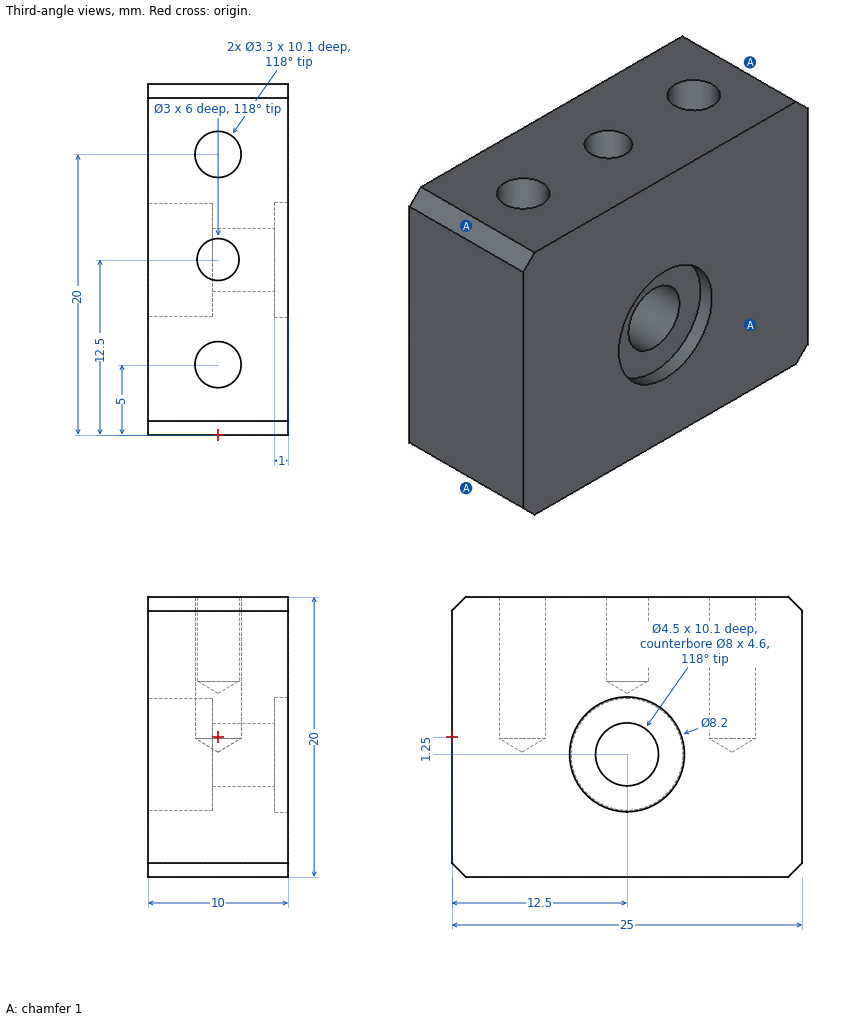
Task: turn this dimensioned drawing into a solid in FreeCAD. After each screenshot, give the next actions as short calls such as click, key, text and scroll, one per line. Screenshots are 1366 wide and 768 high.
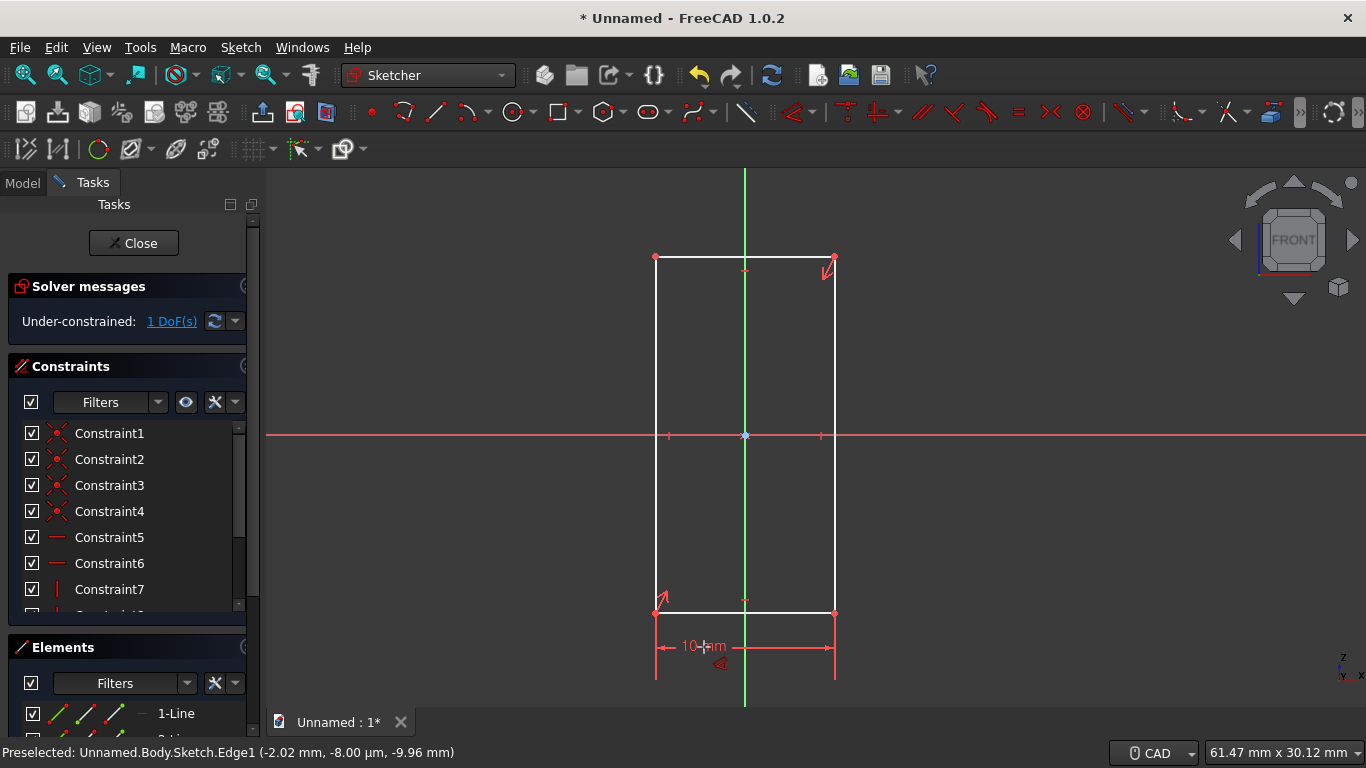
click(835, 506)
click(869, 353)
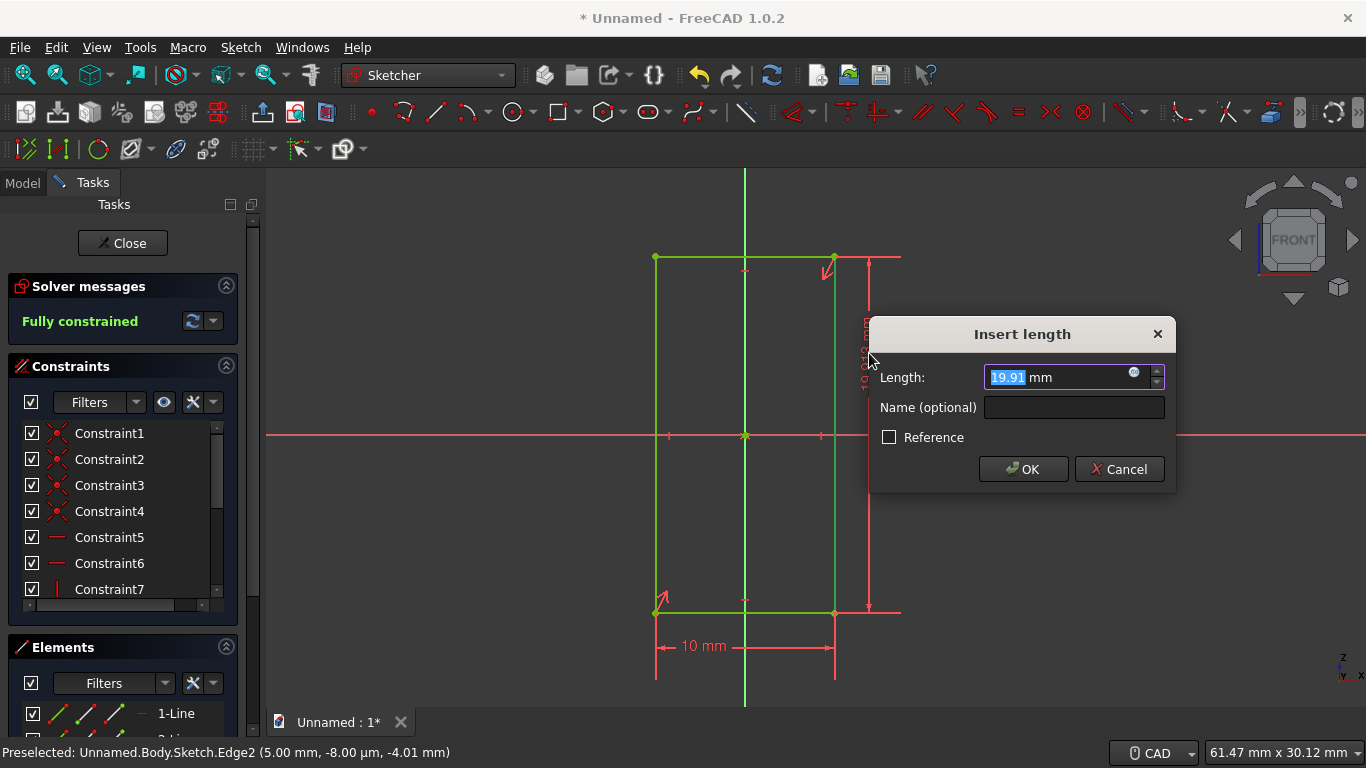
text(20)
key(Return)
key(Escape)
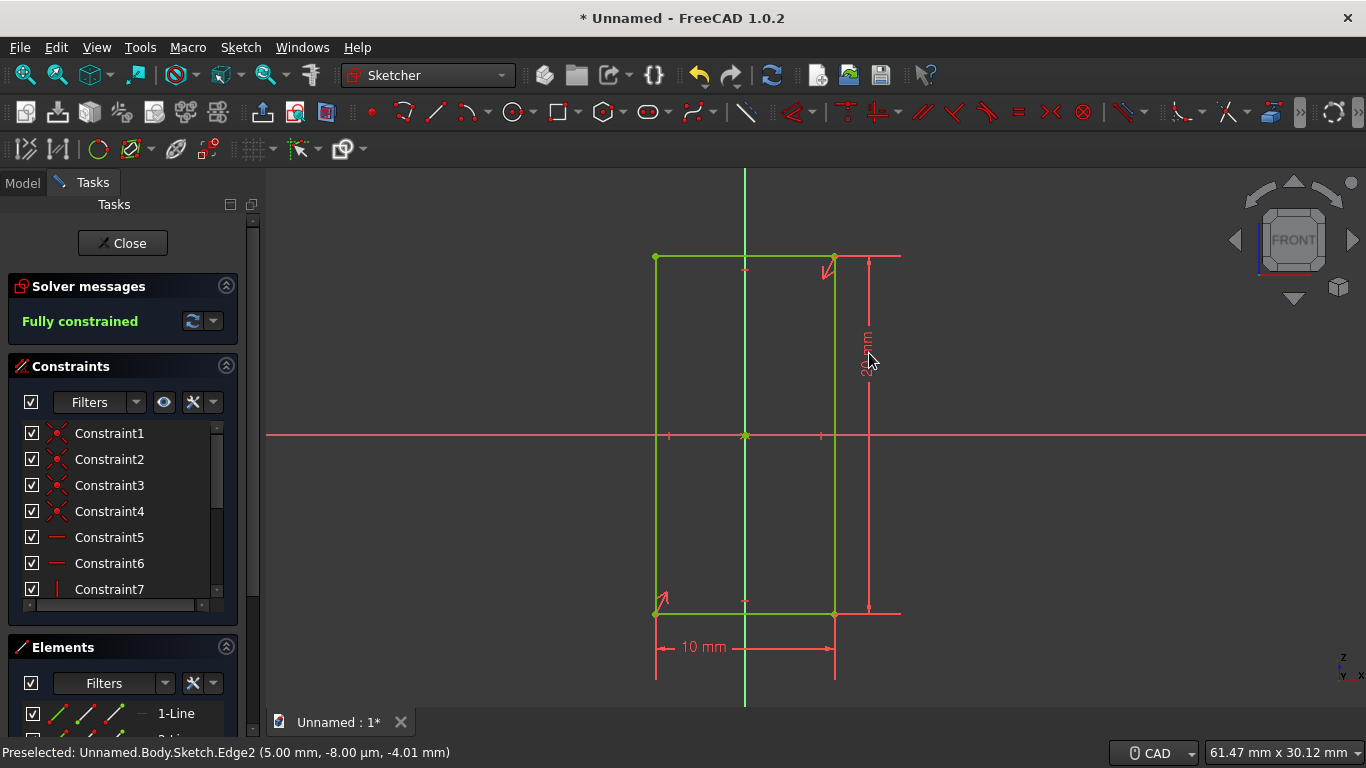
click(123, 243)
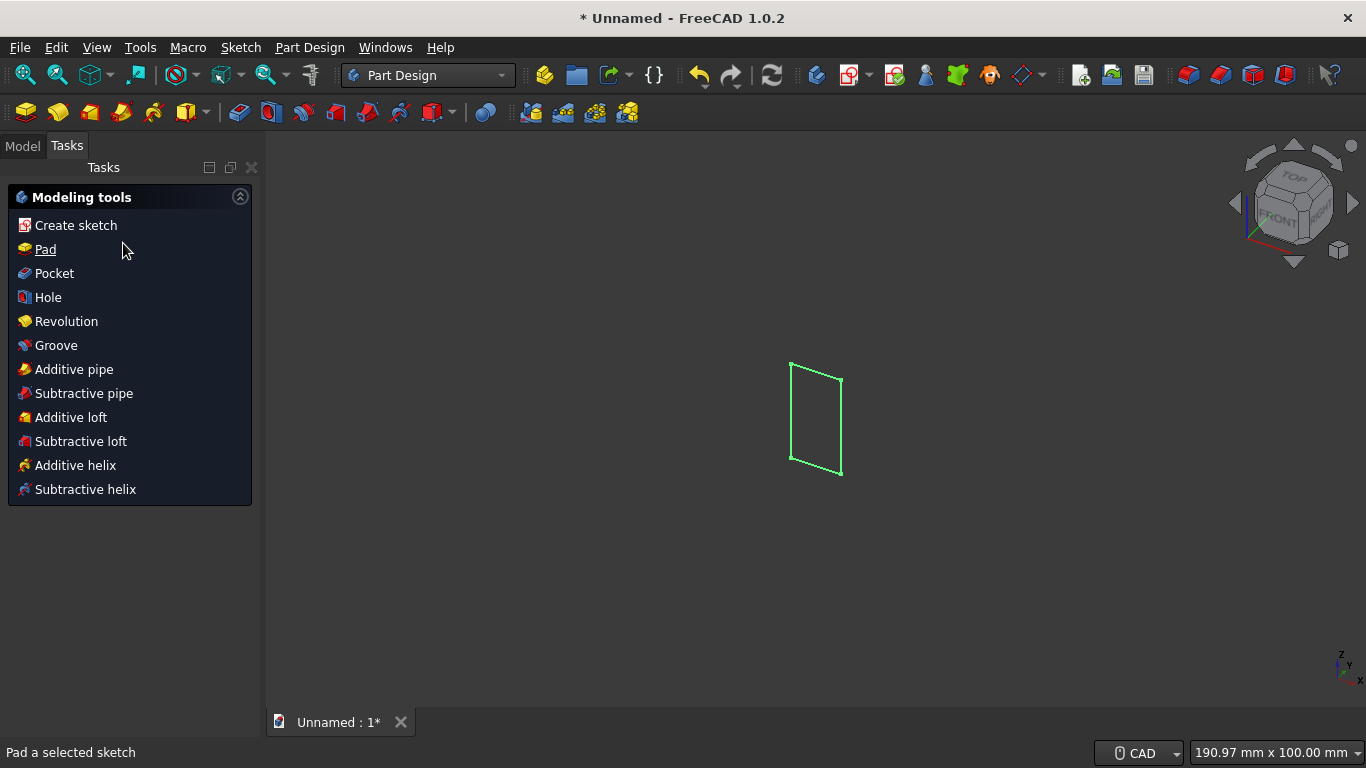
click(26, 112)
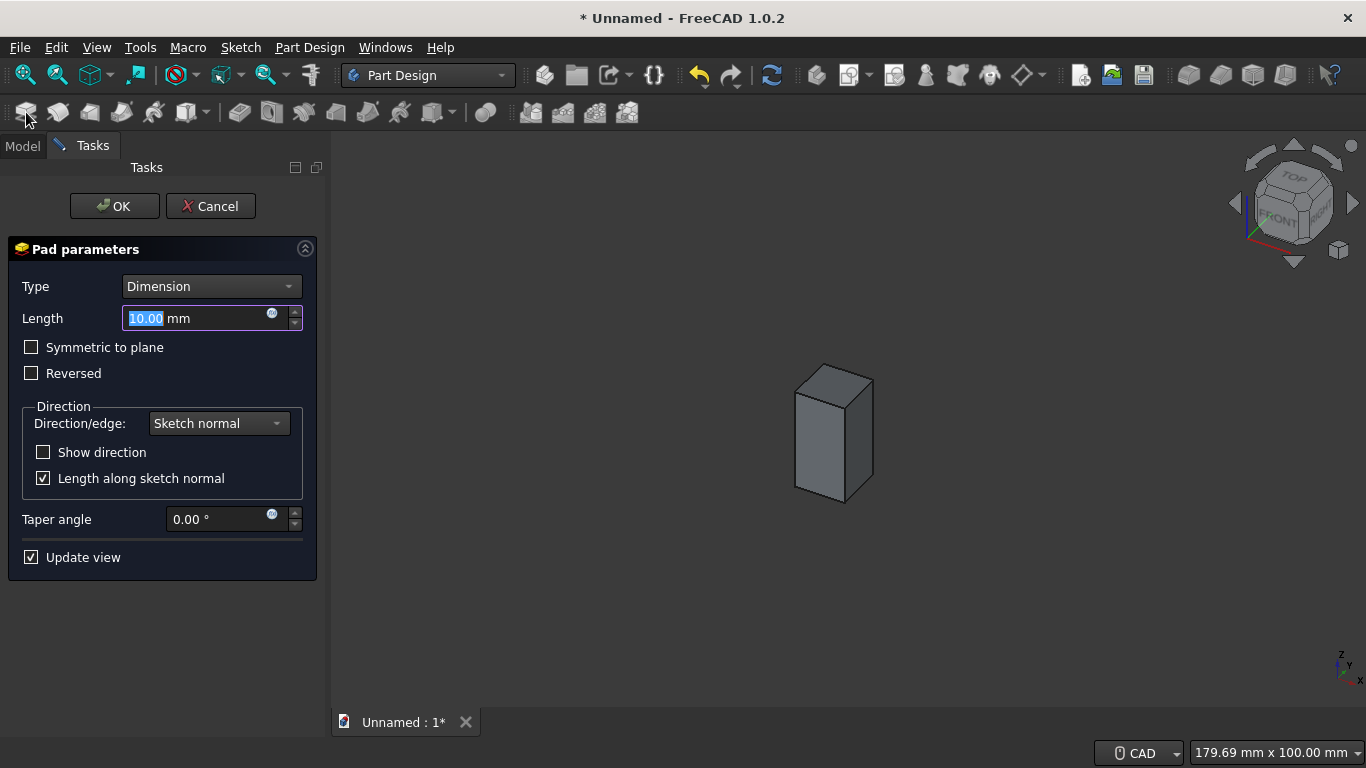
text(25)
key(Tab)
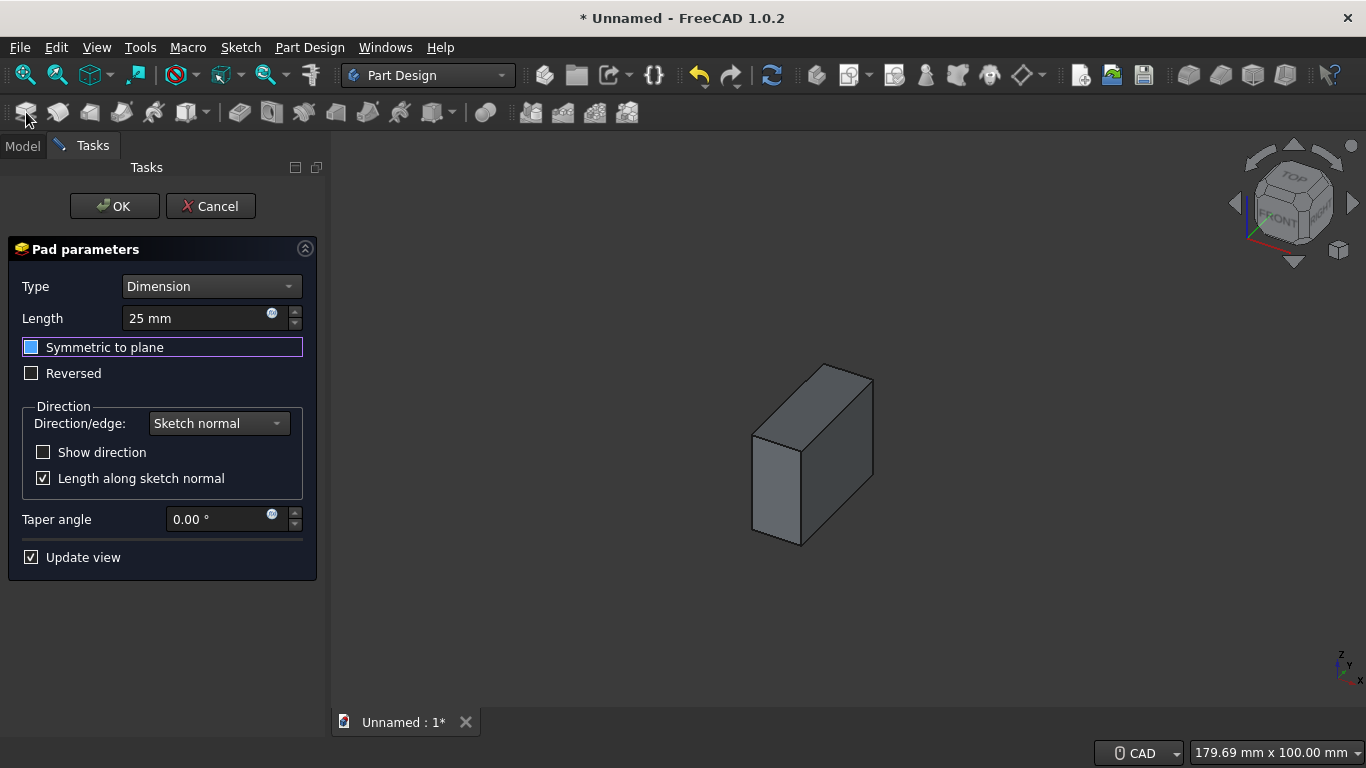
click(30, 373)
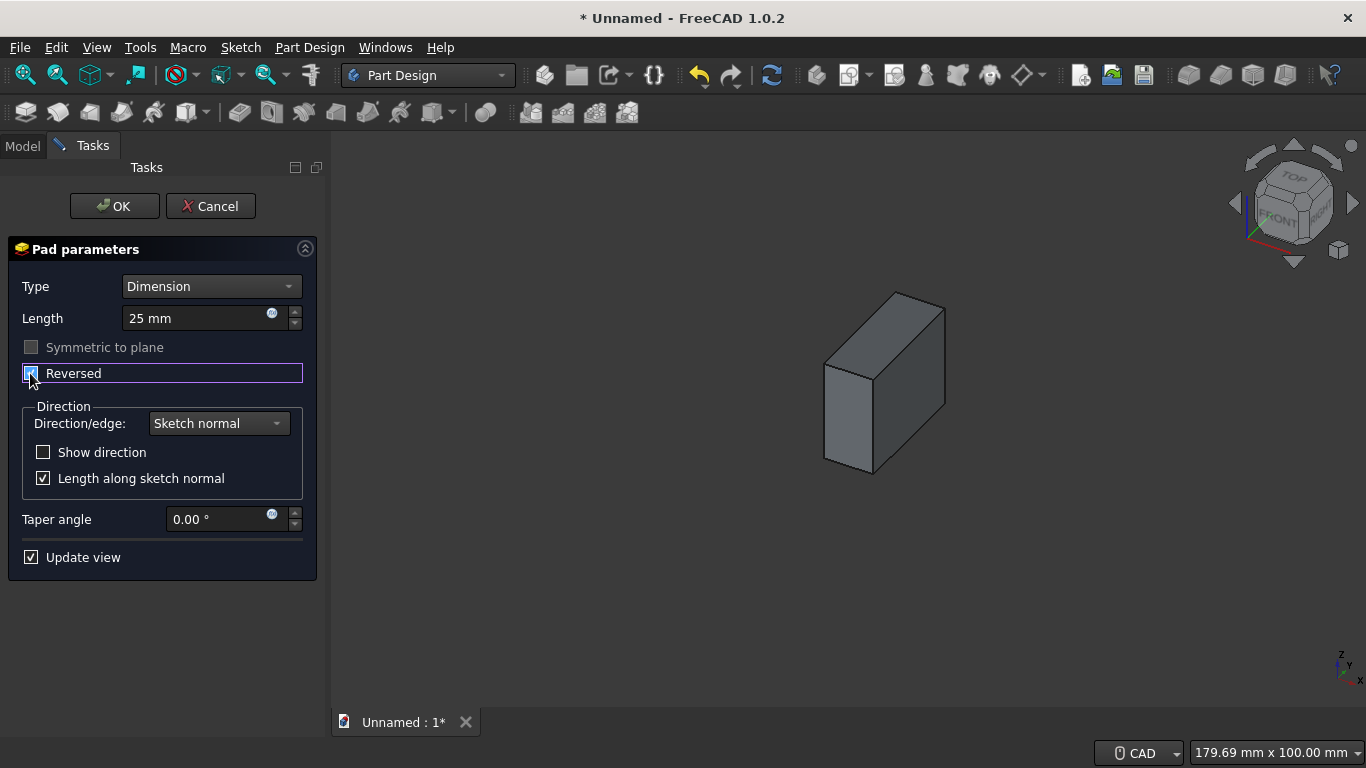
click(115, 206)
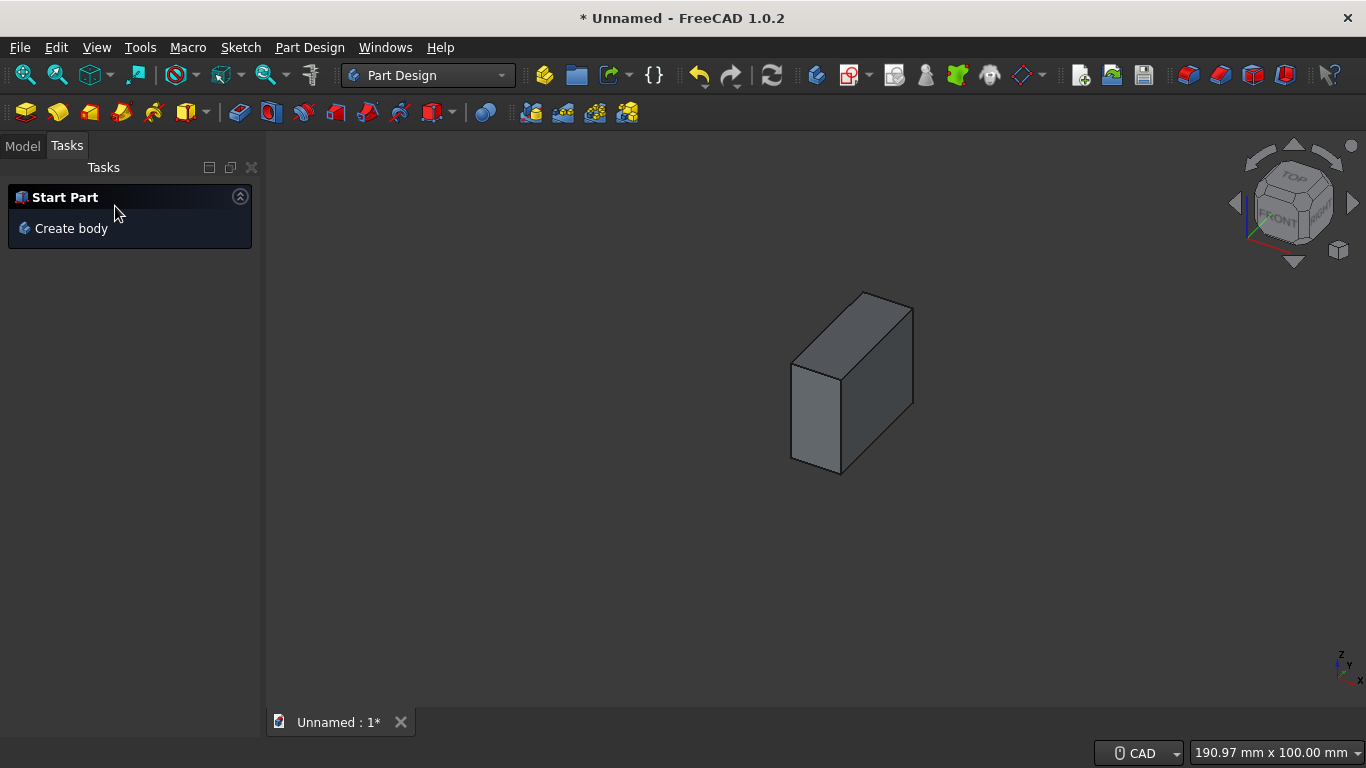
click(26, 76)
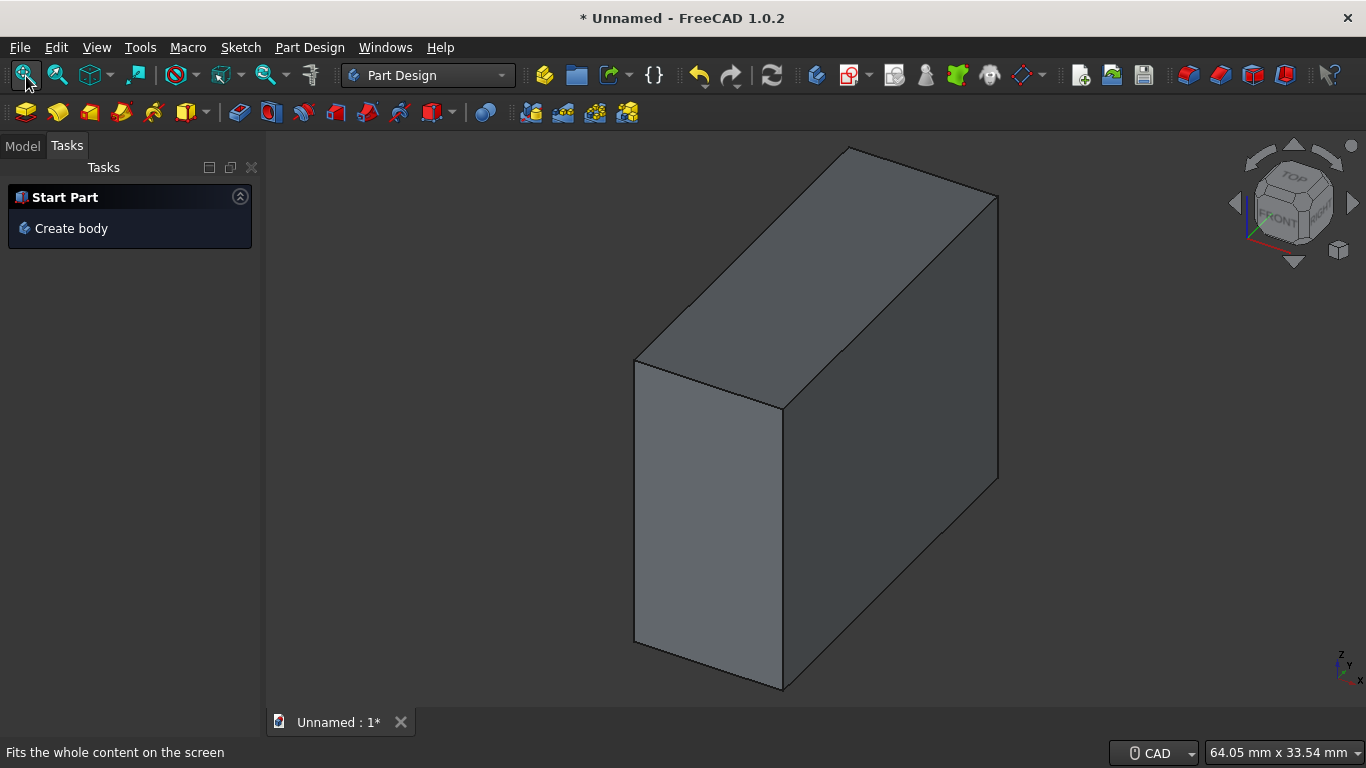
key(6)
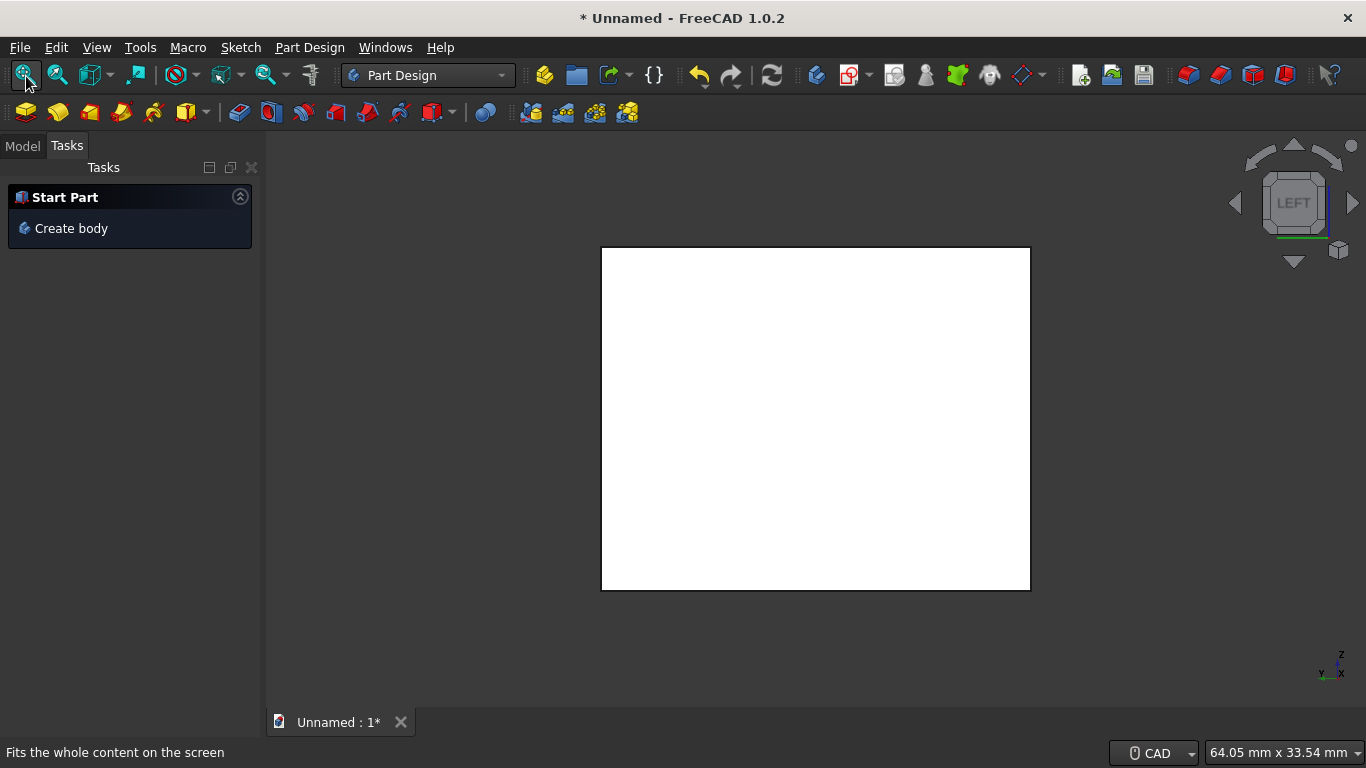
click(816, 418)